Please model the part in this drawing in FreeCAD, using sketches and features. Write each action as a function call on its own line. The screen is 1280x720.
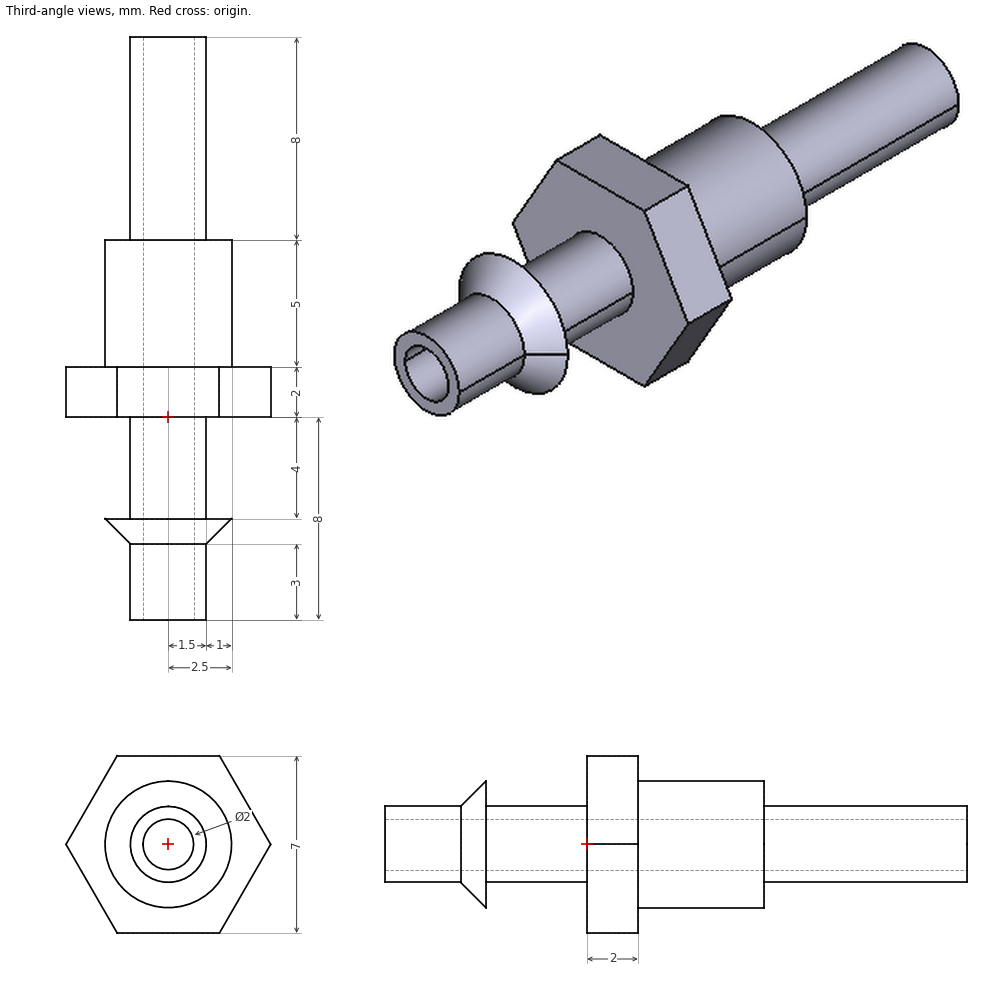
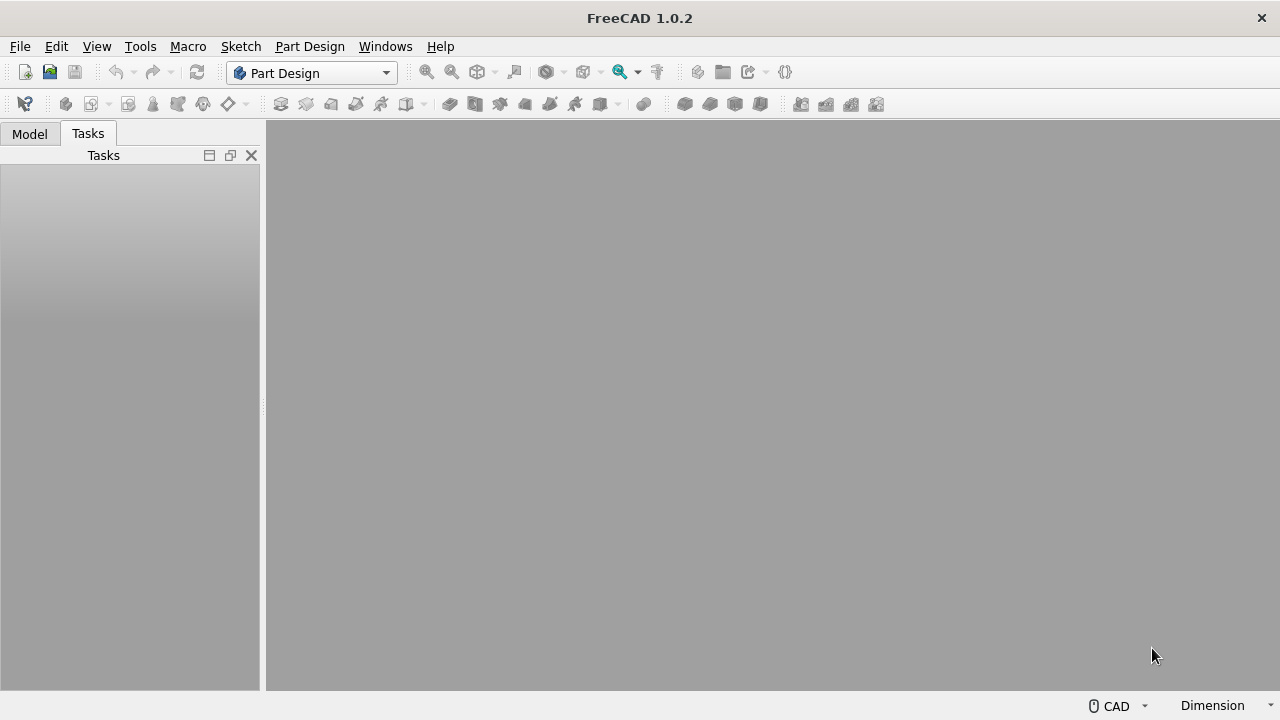
click(25, 72)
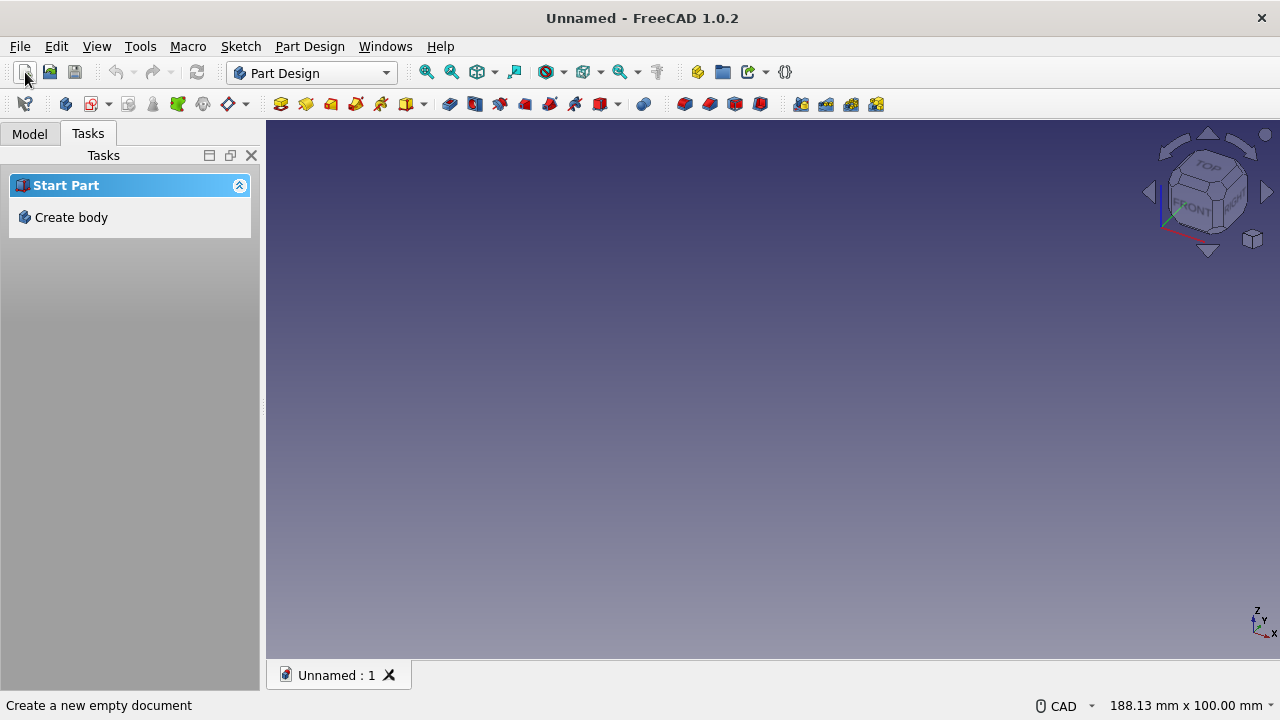
click(90, 104)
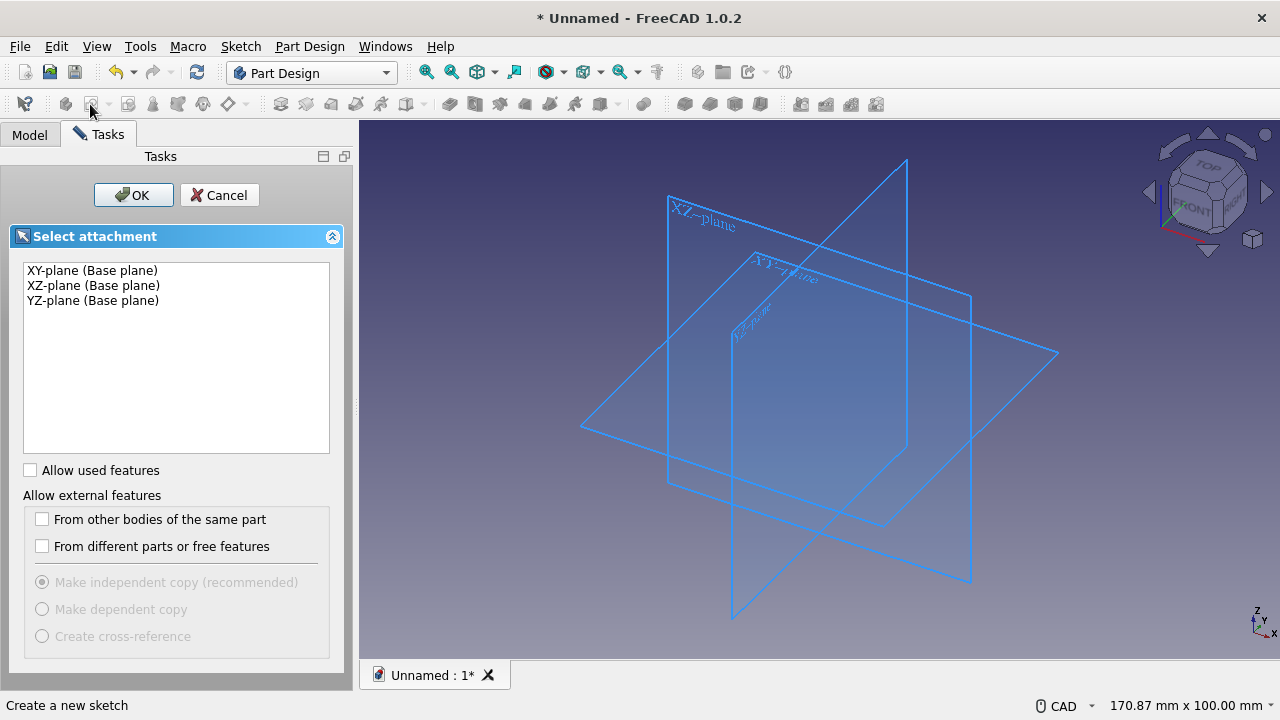
click(84, 270)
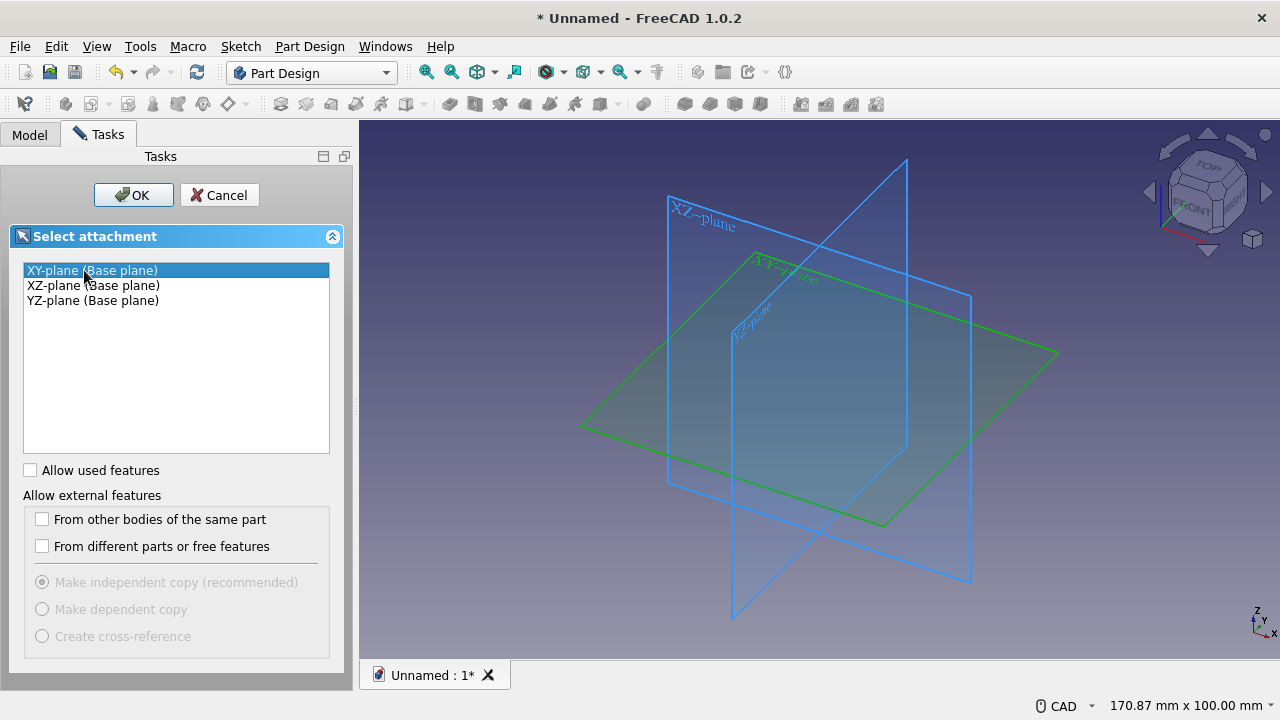
click(134, 195)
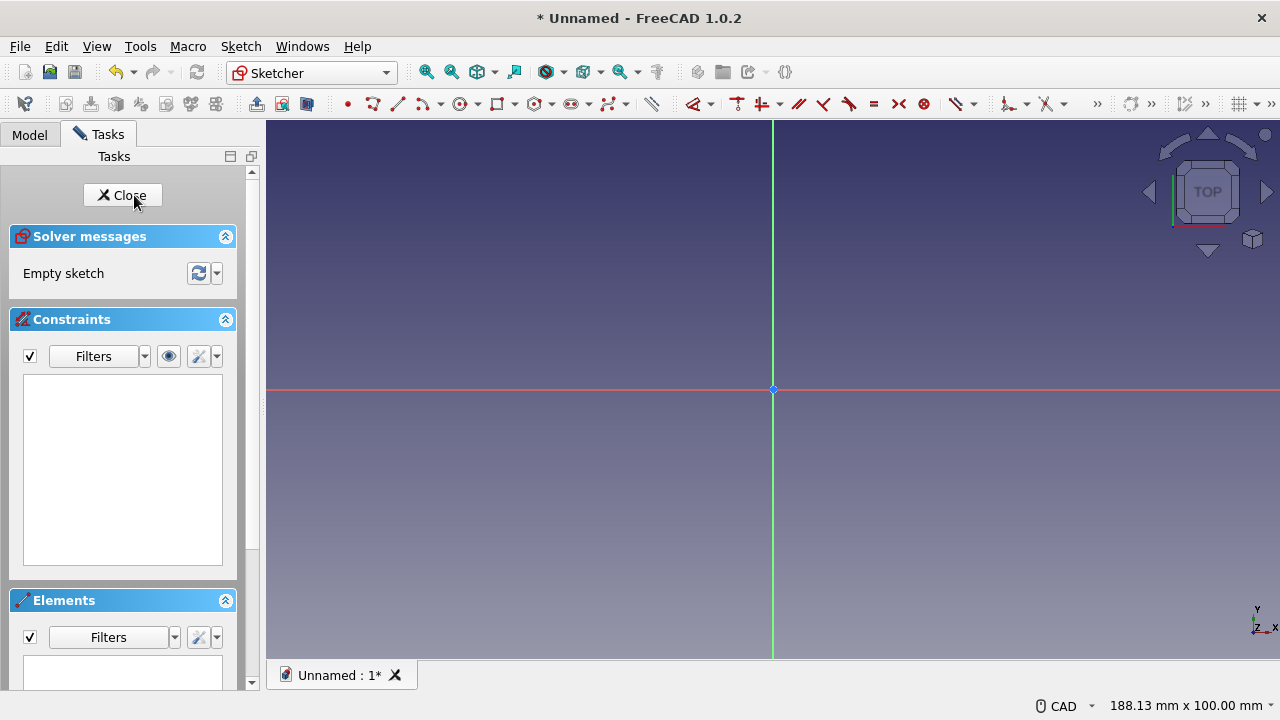
scroll(792, 414, up, 10)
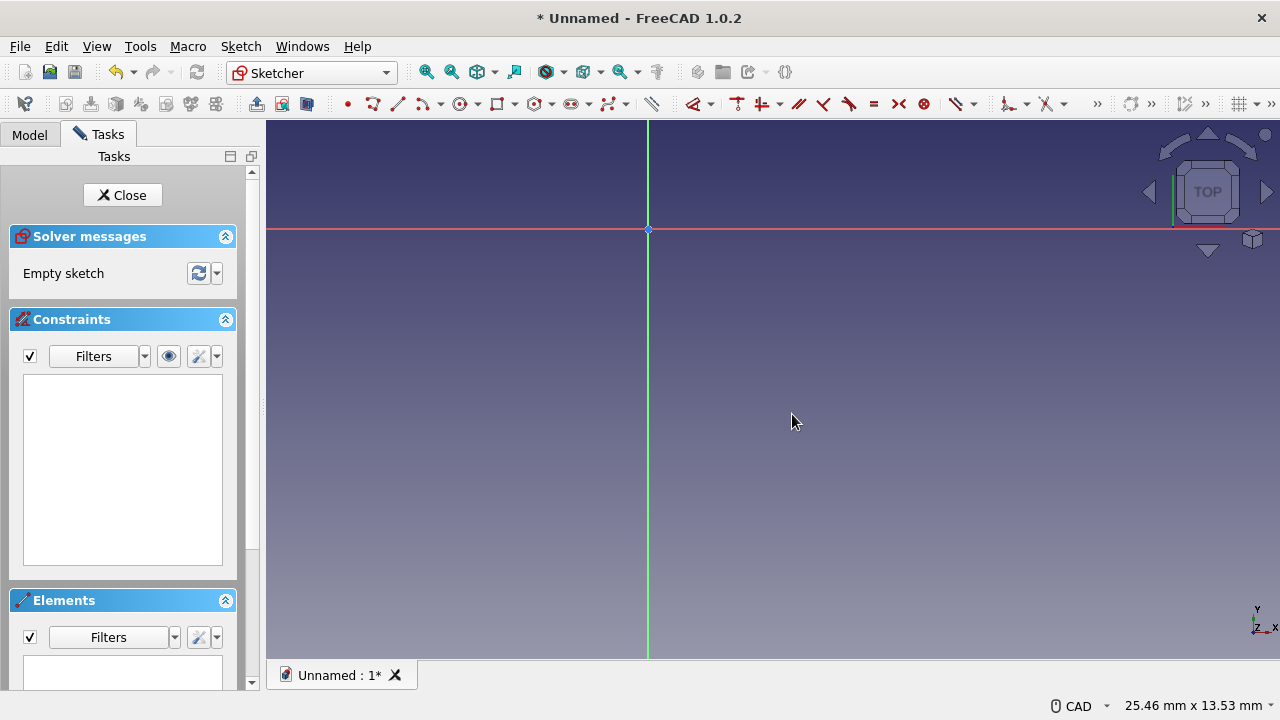
key(g)
key(m)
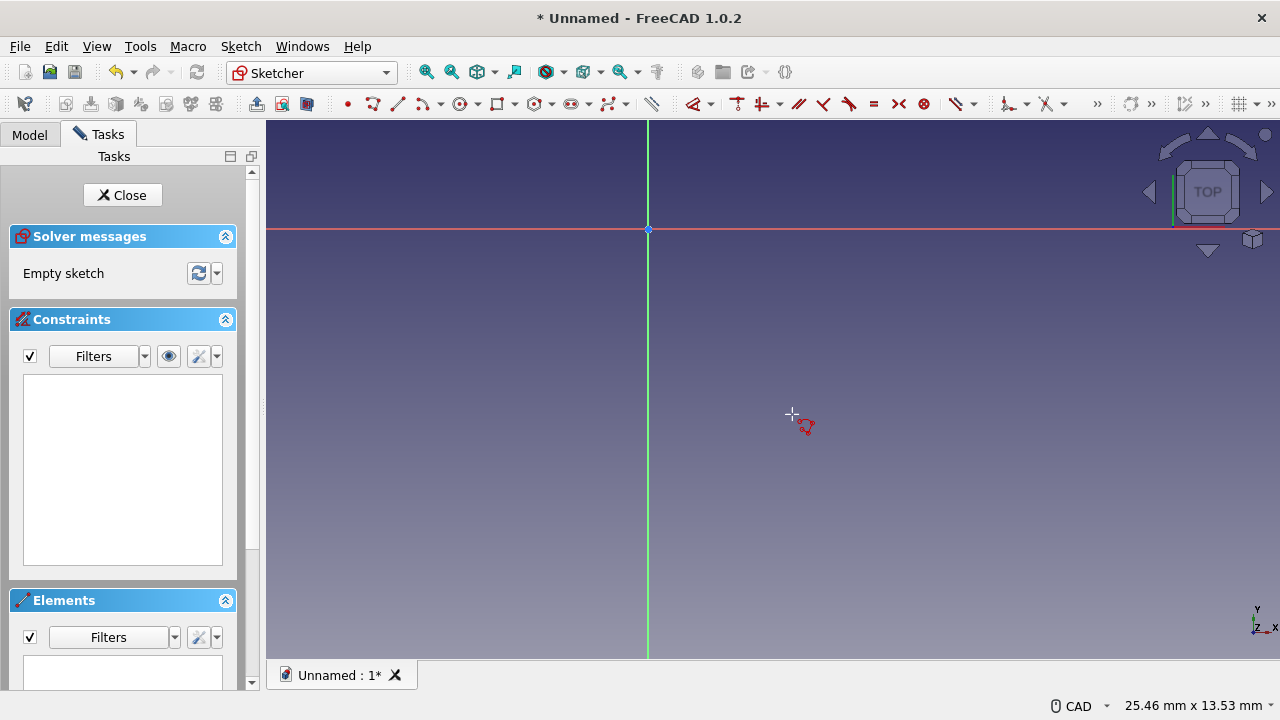
click(648, 229)
click(657, 548)
click(708, 548)
click(708, 429)
click(748, 389)
click(708, 389)
click(708, 238)
click(648, 229)
key(Escape)
key(Escape)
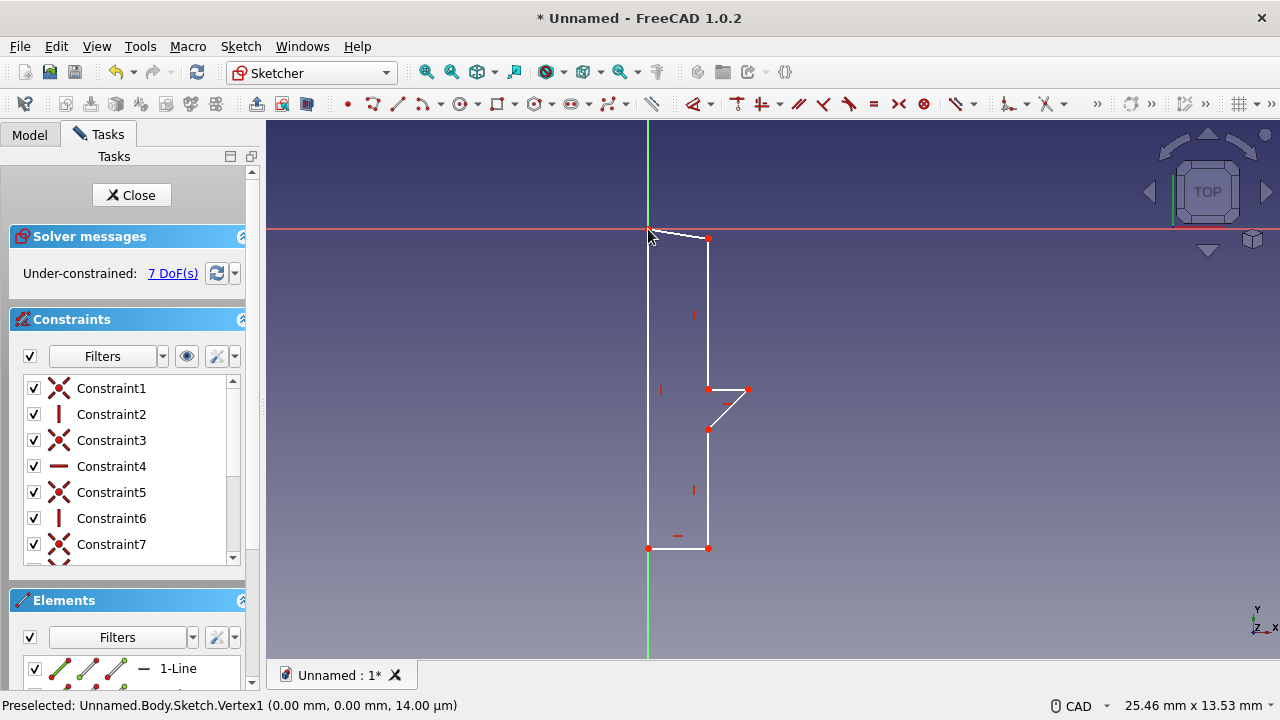
click(666, 232)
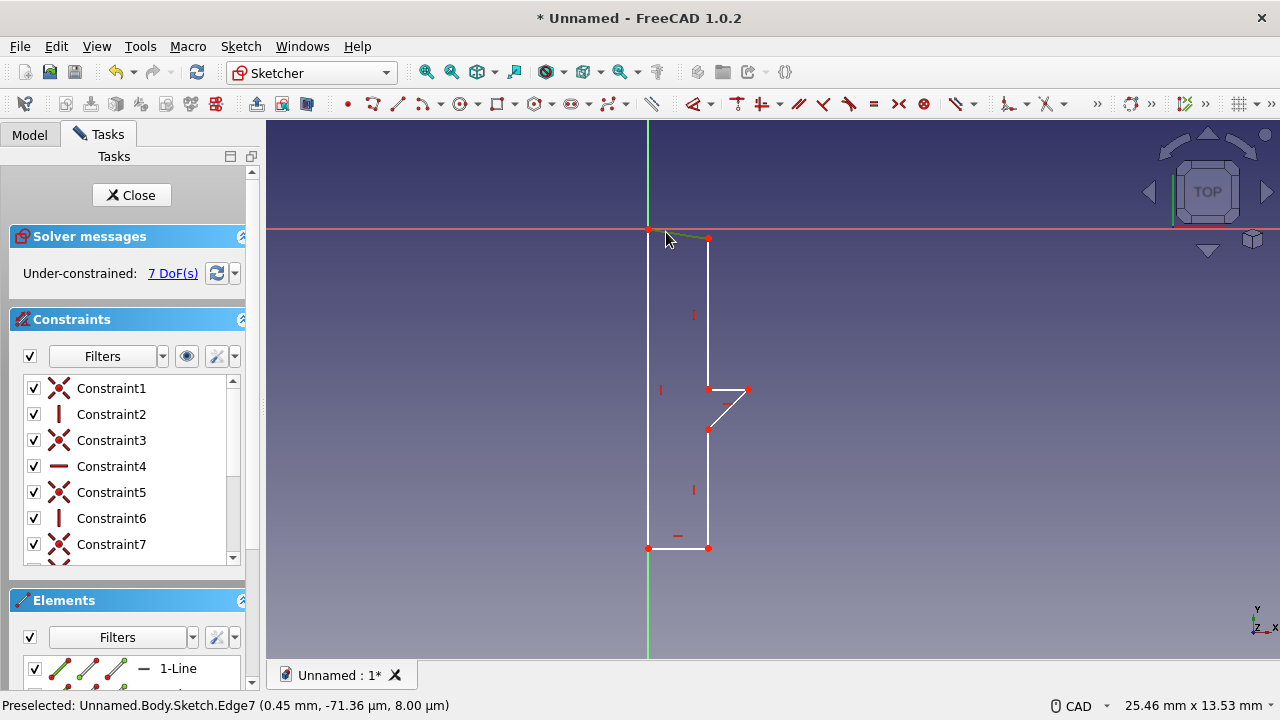
key(h)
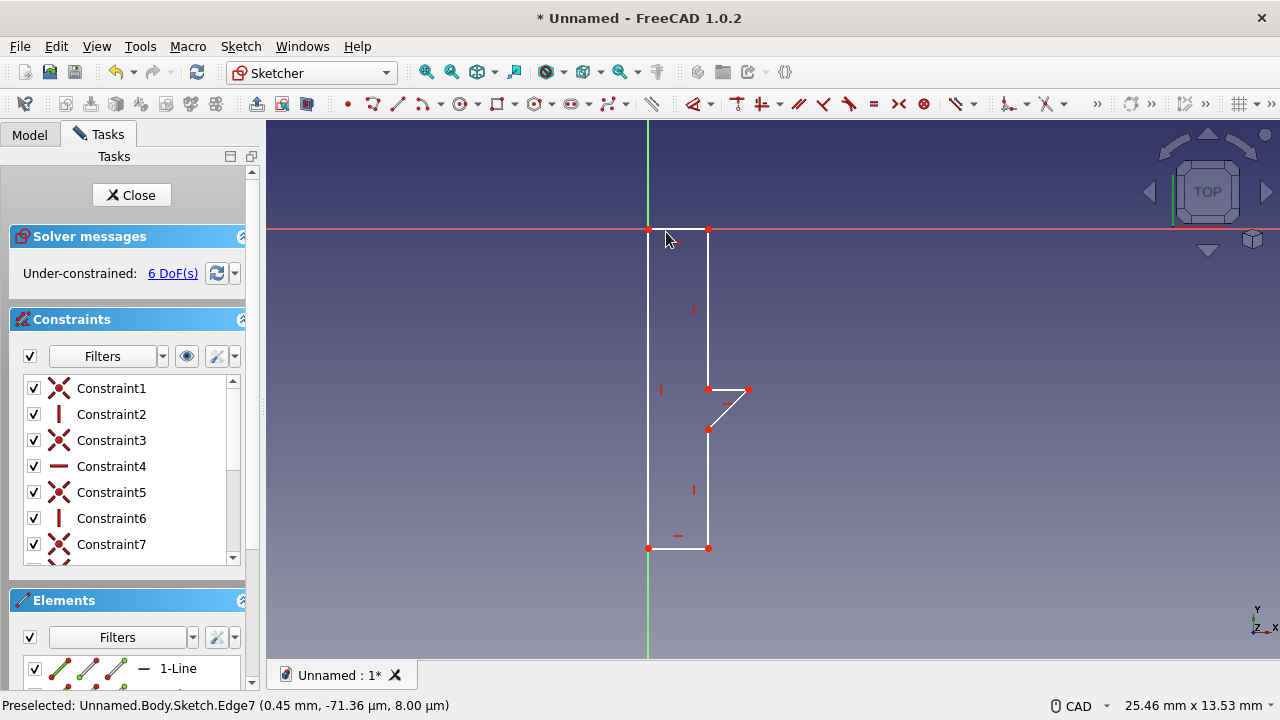
click(692, 104)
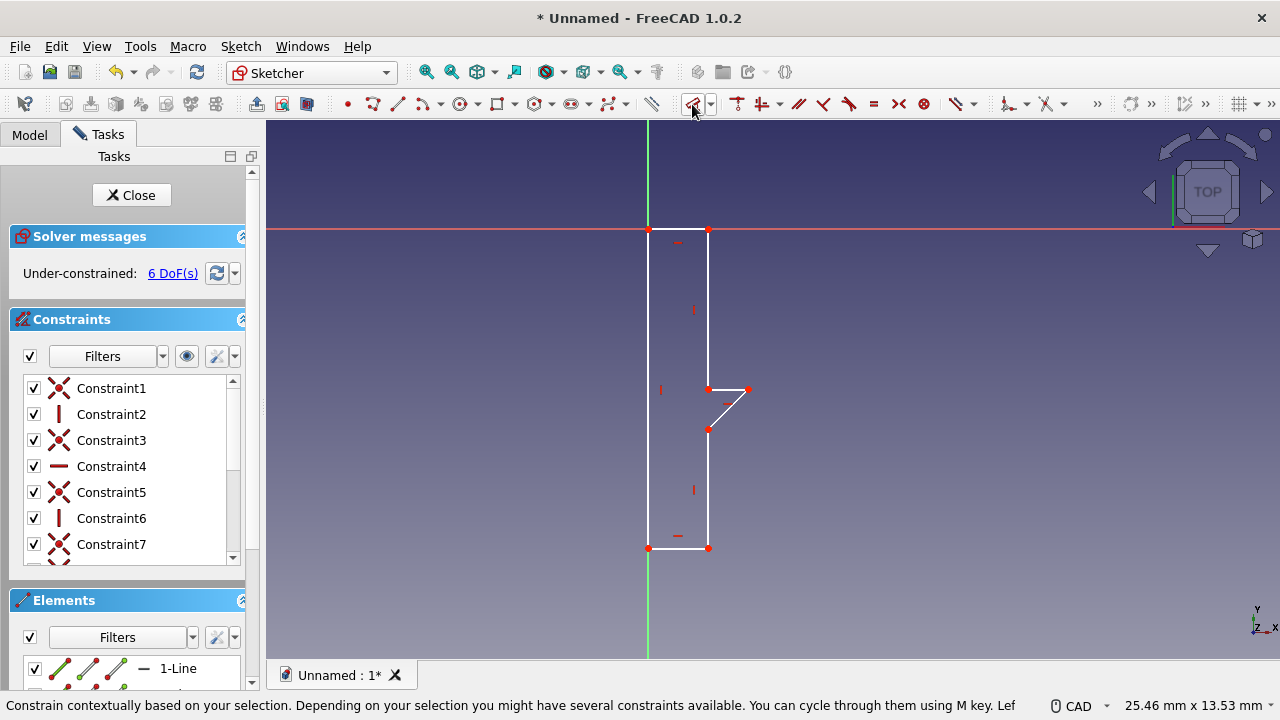
click(648, 325)
click(614, 389)